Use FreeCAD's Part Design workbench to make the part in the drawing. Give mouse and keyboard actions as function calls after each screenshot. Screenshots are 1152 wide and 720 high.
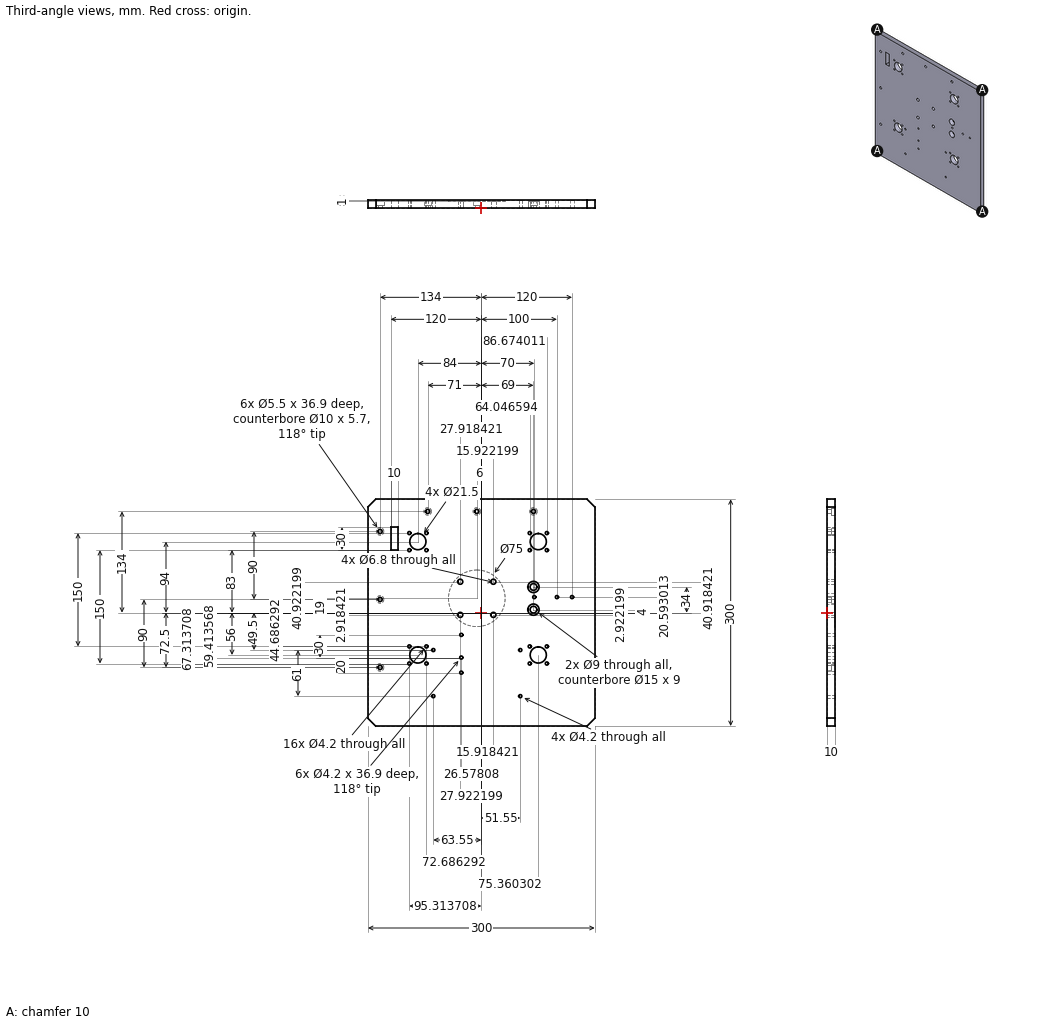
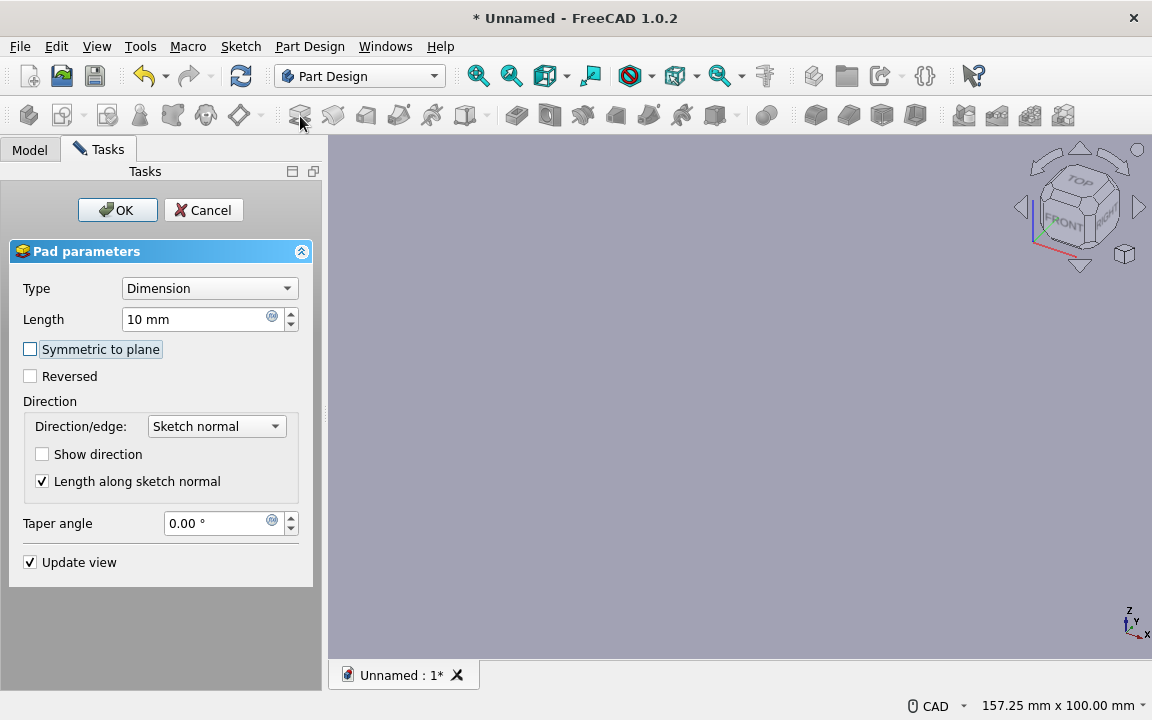
click(31, 376)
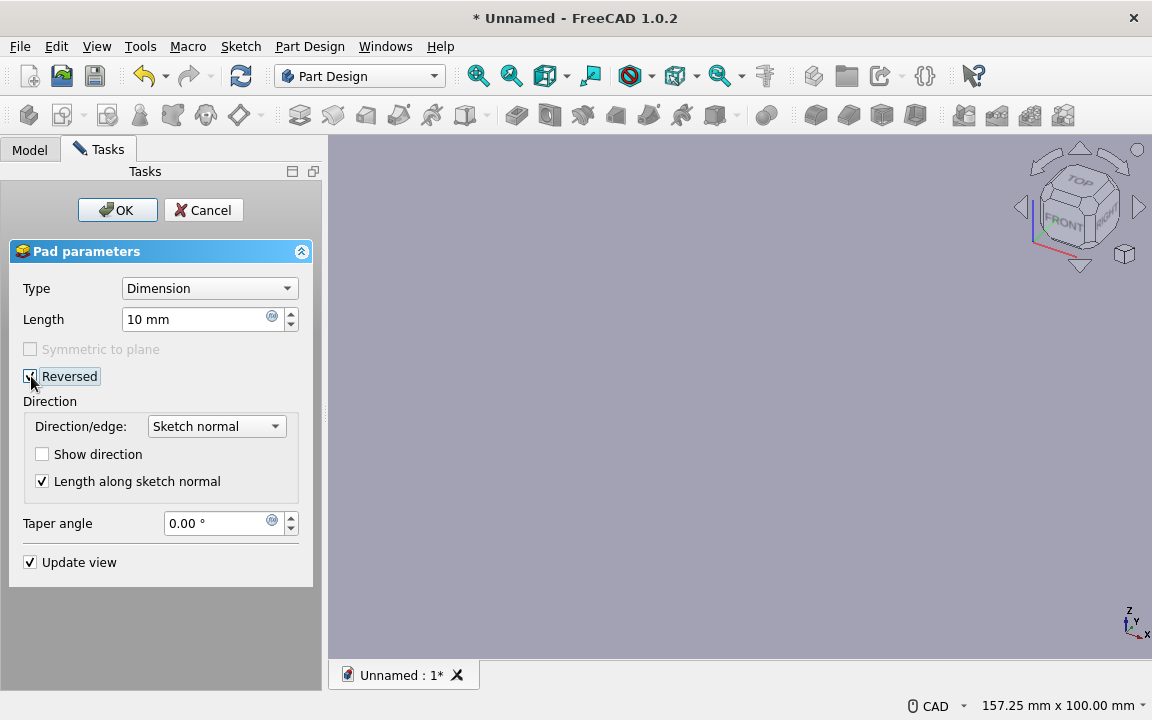
click(118, 210)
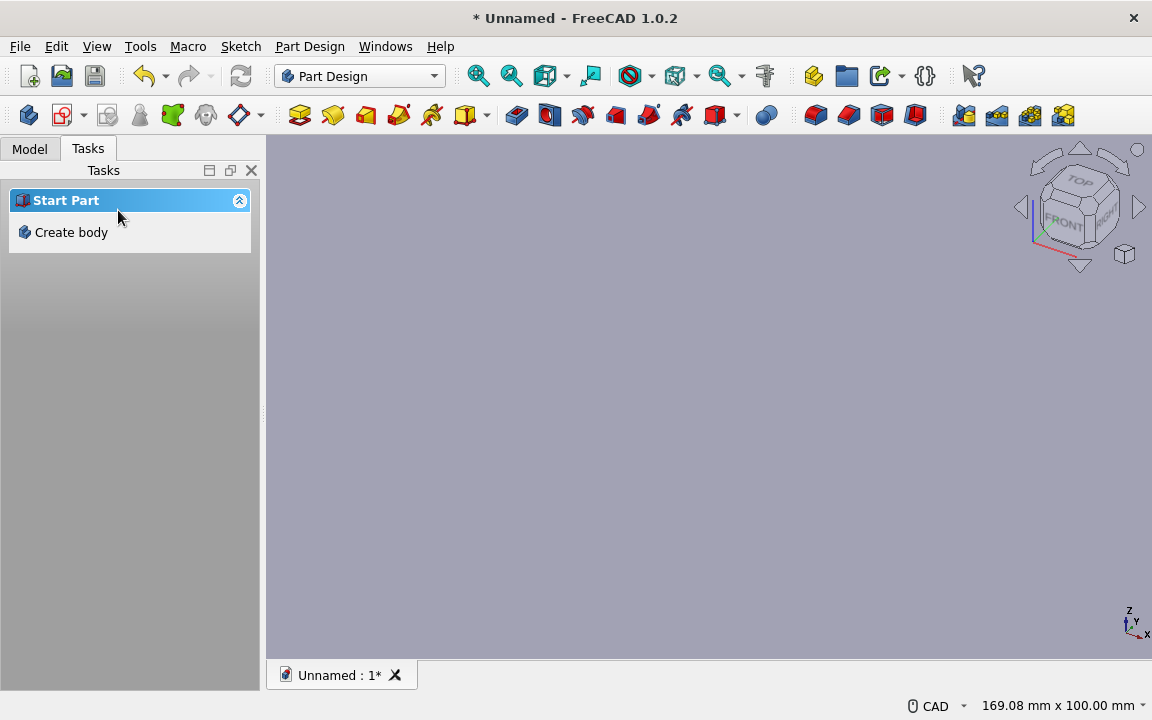
key(v)
key(f)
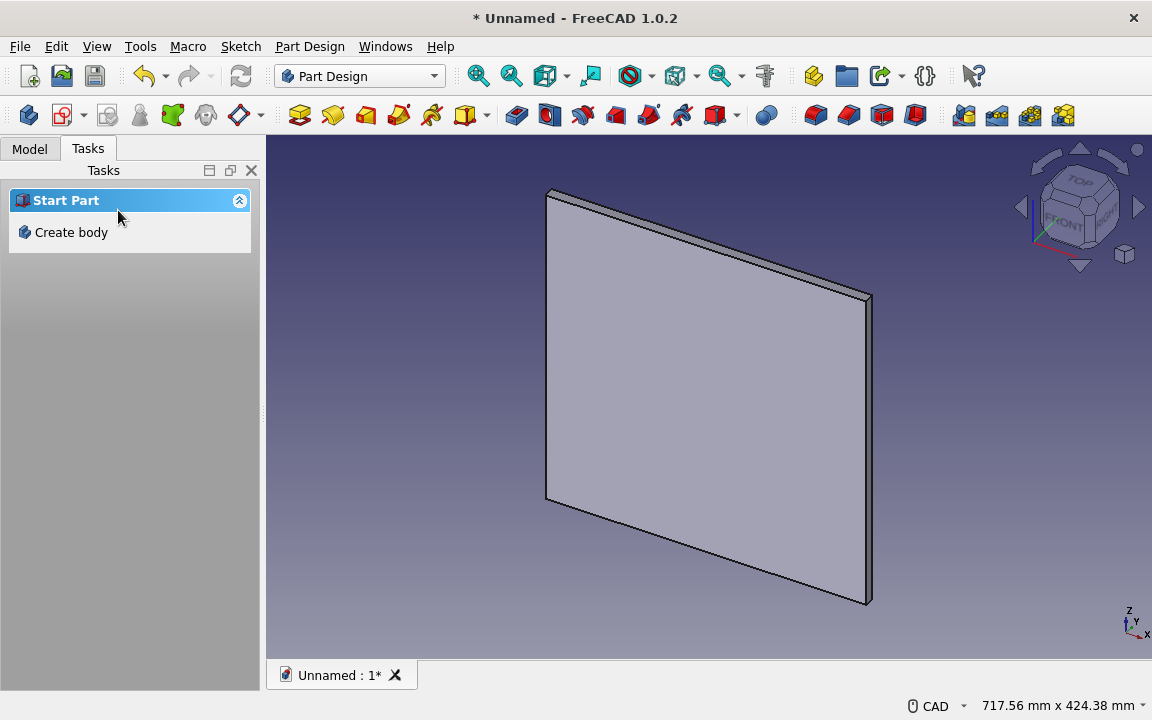
key(4)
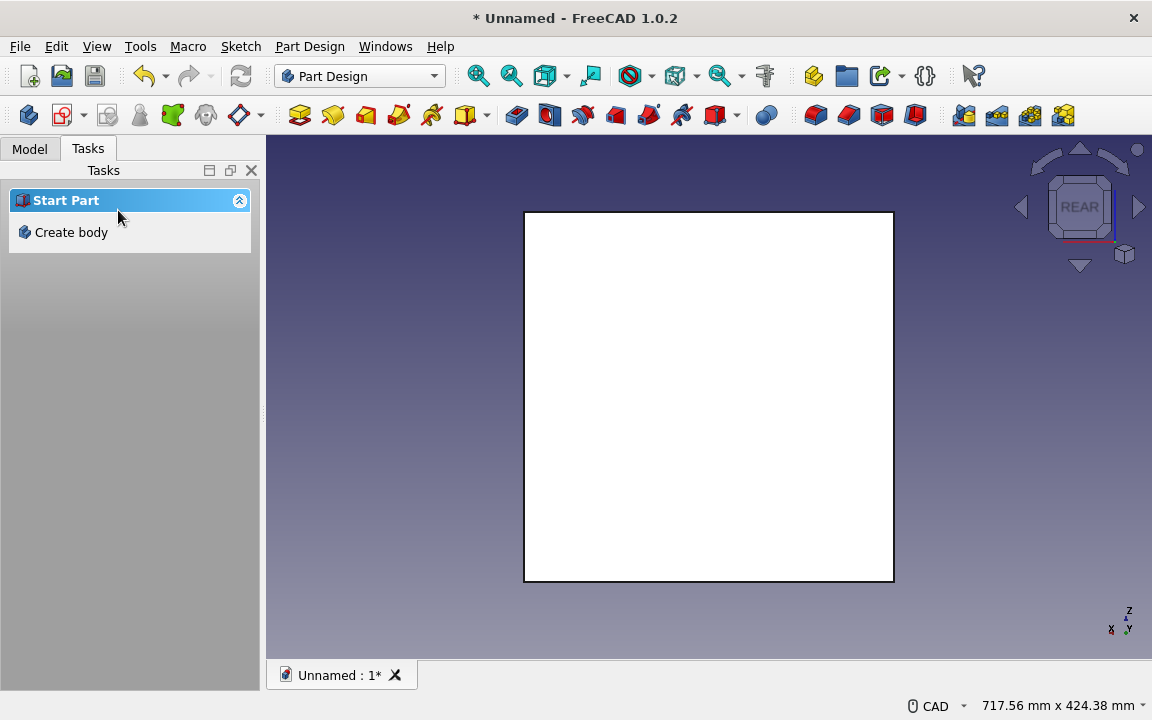
click(709, 396)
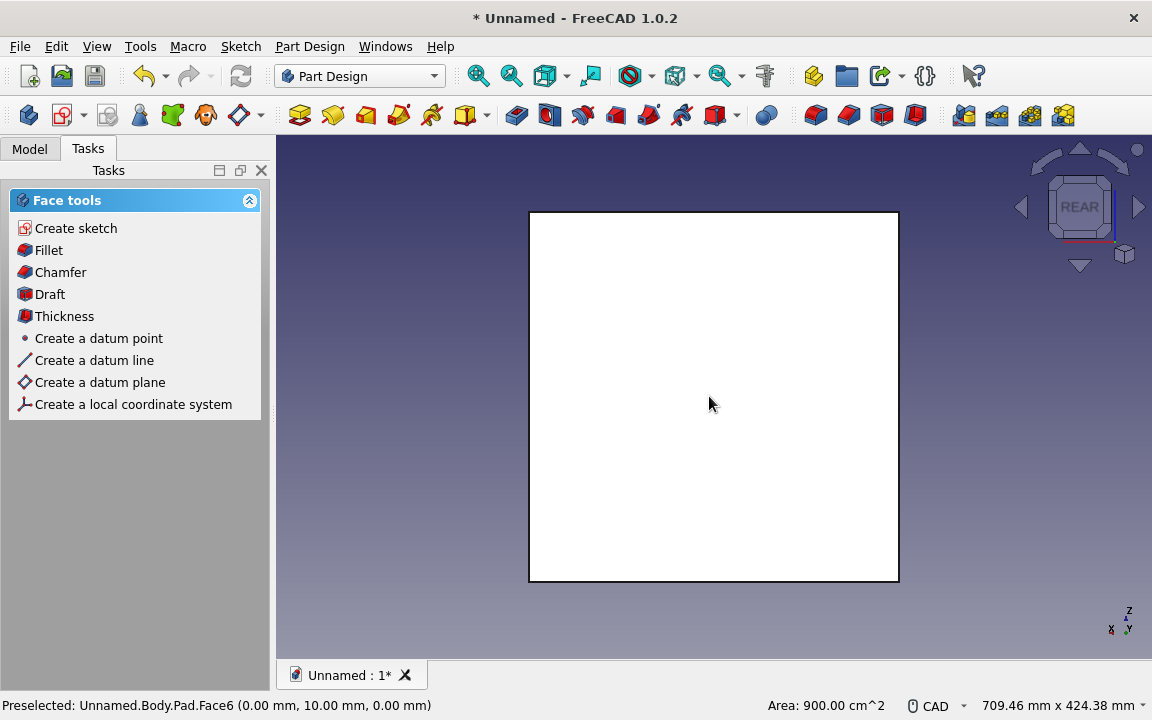
click(62, 116)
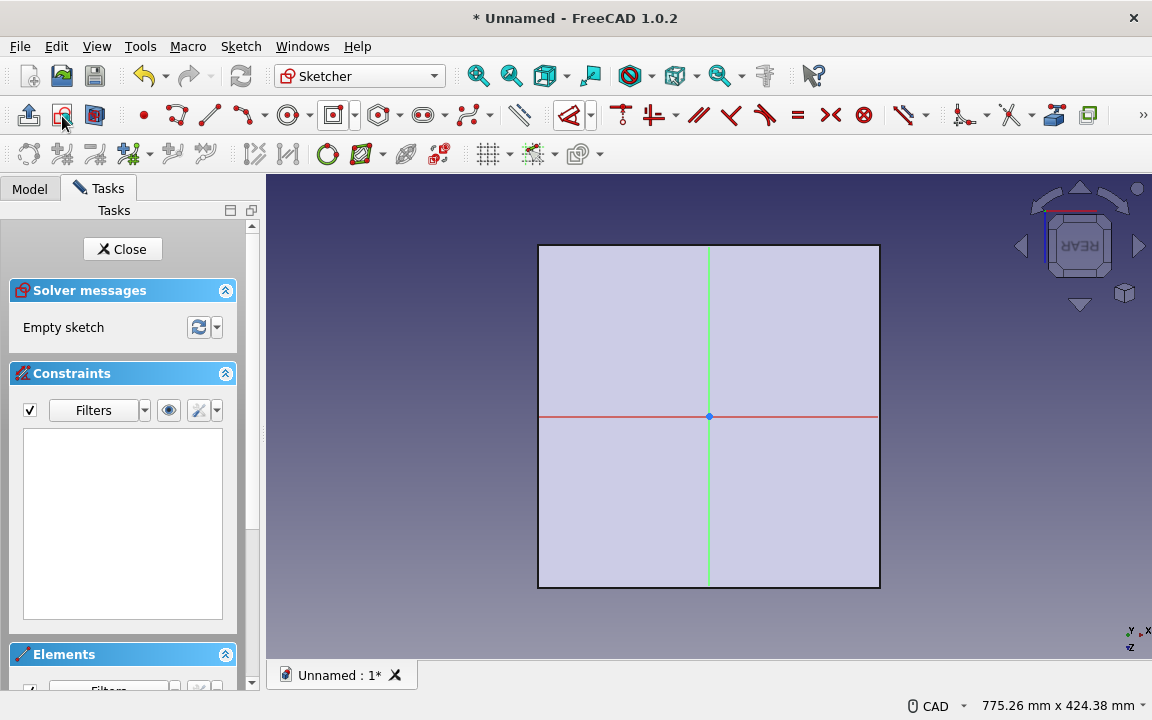
scroll(729, 448, up, 6)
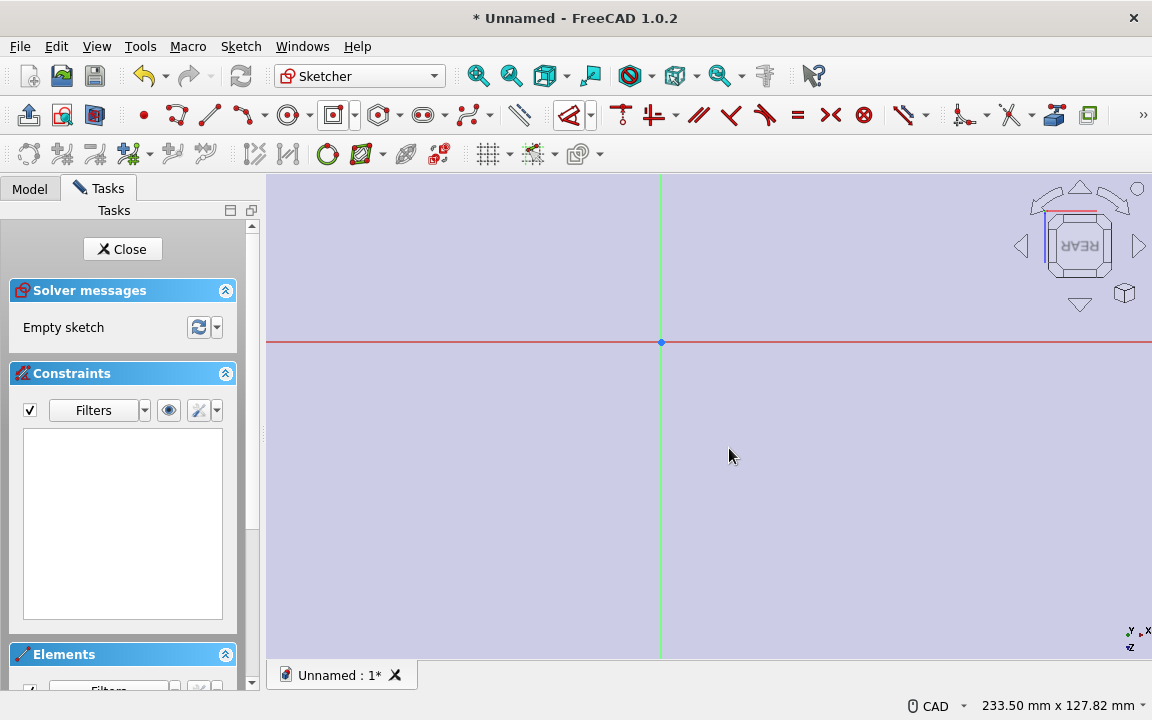
click(288, 116)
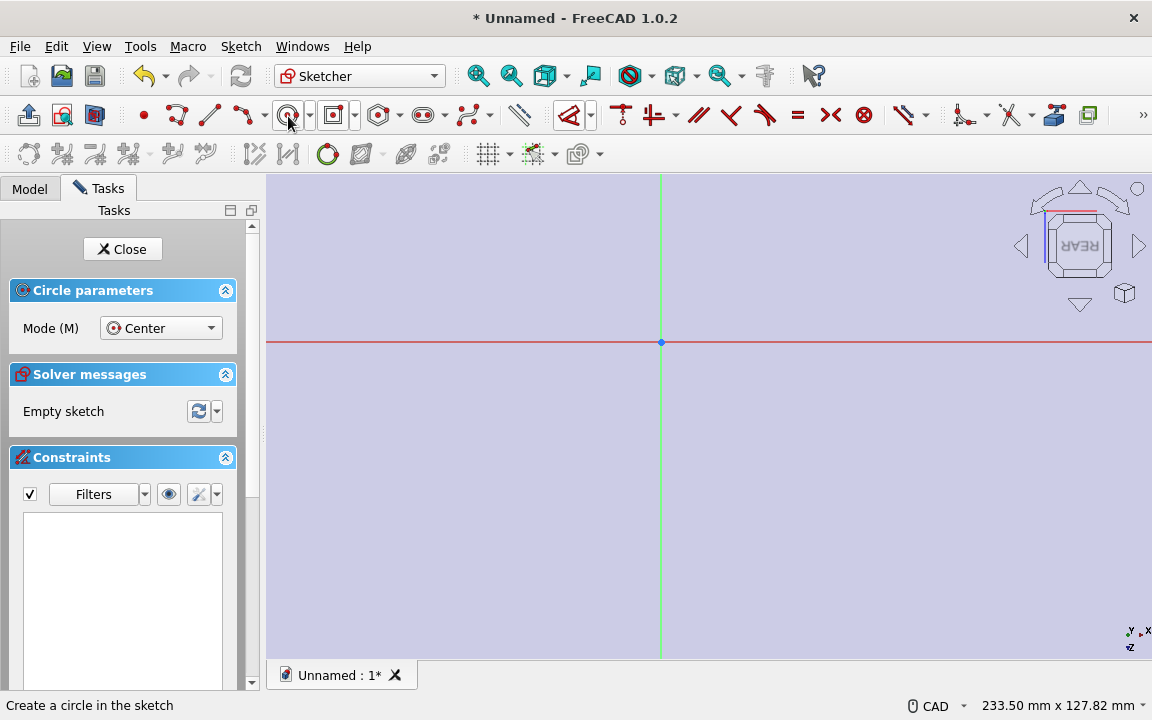
click(639, 414)
move(739, 314)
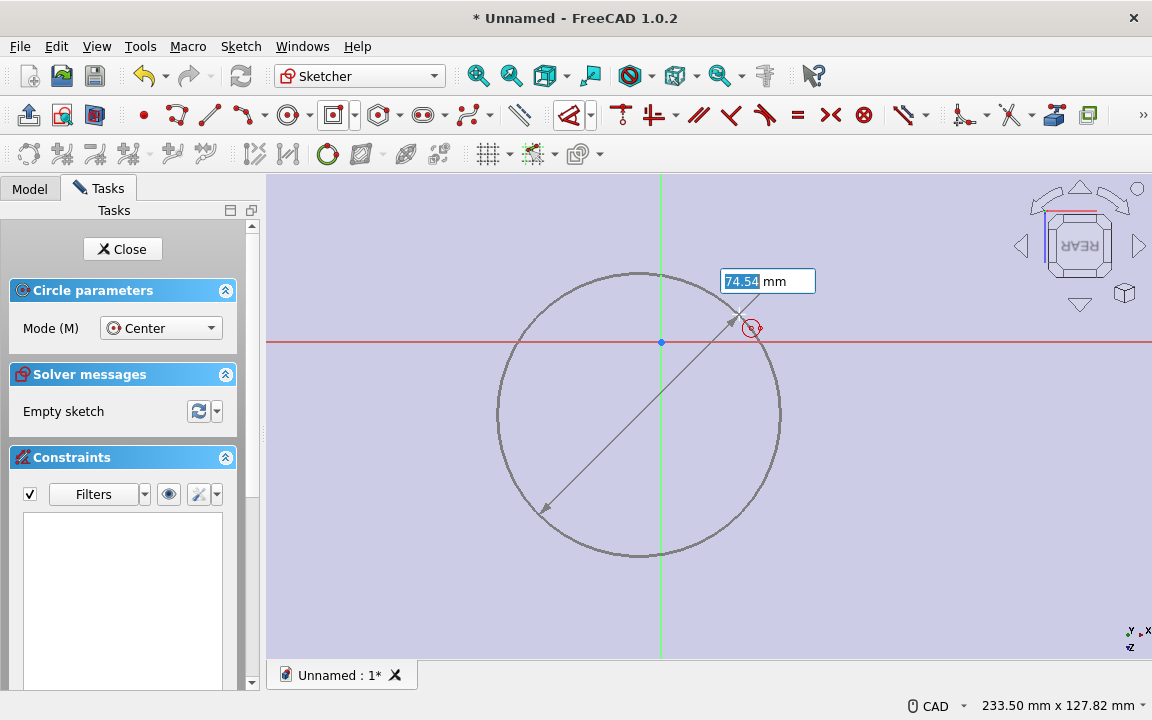
text(75)
key(Return)
key(Escape)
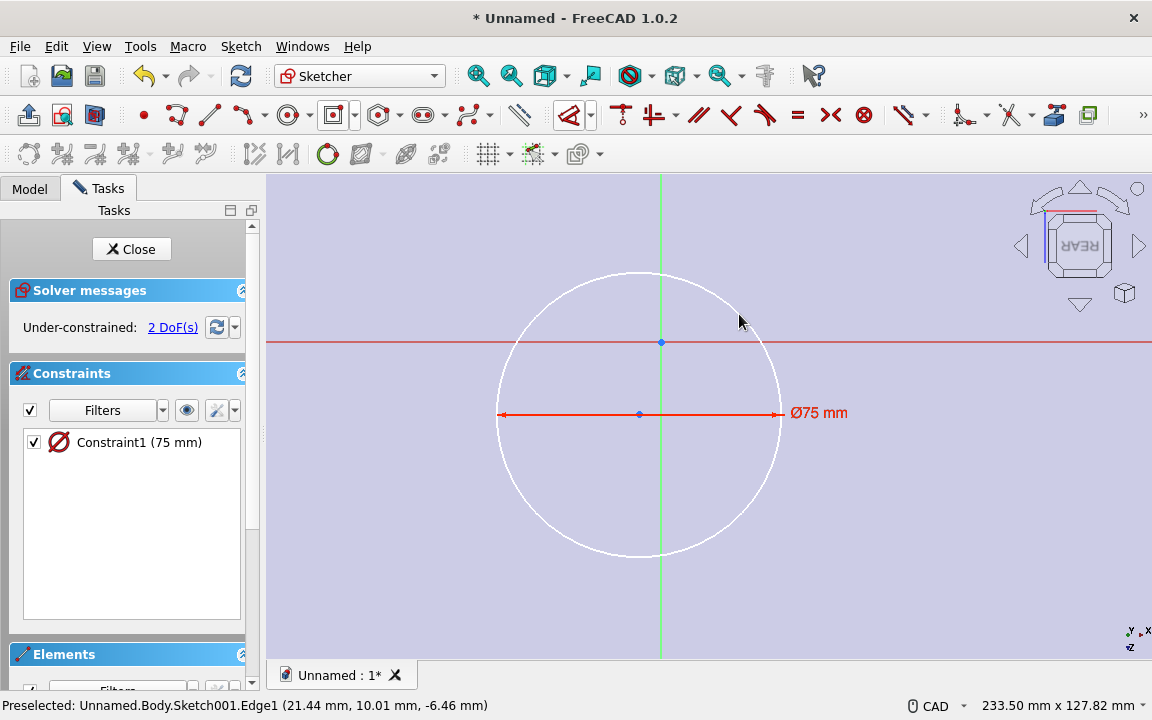
scroll(639, 415, up, 3)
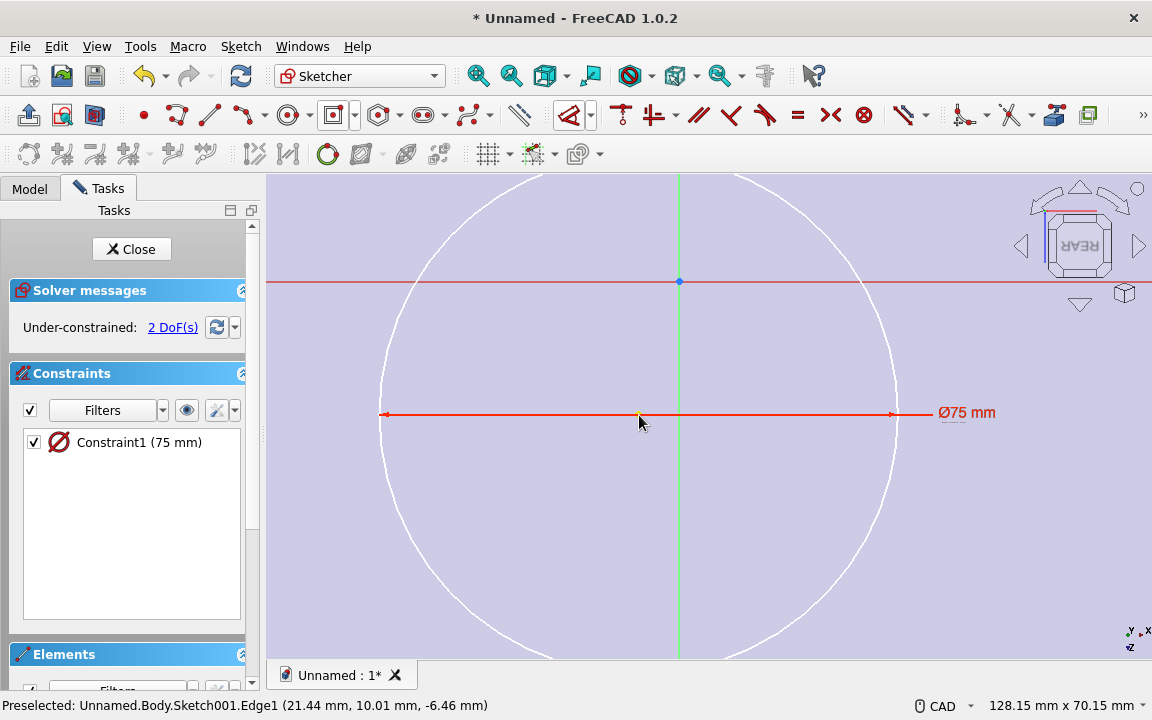
click(639, 415)